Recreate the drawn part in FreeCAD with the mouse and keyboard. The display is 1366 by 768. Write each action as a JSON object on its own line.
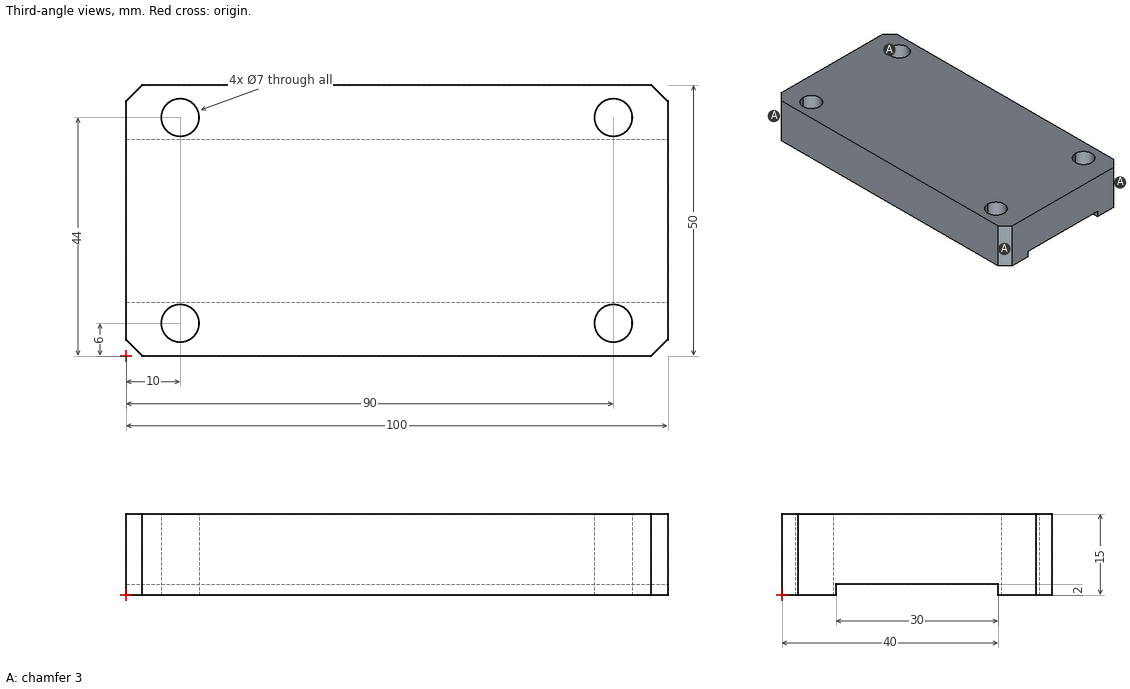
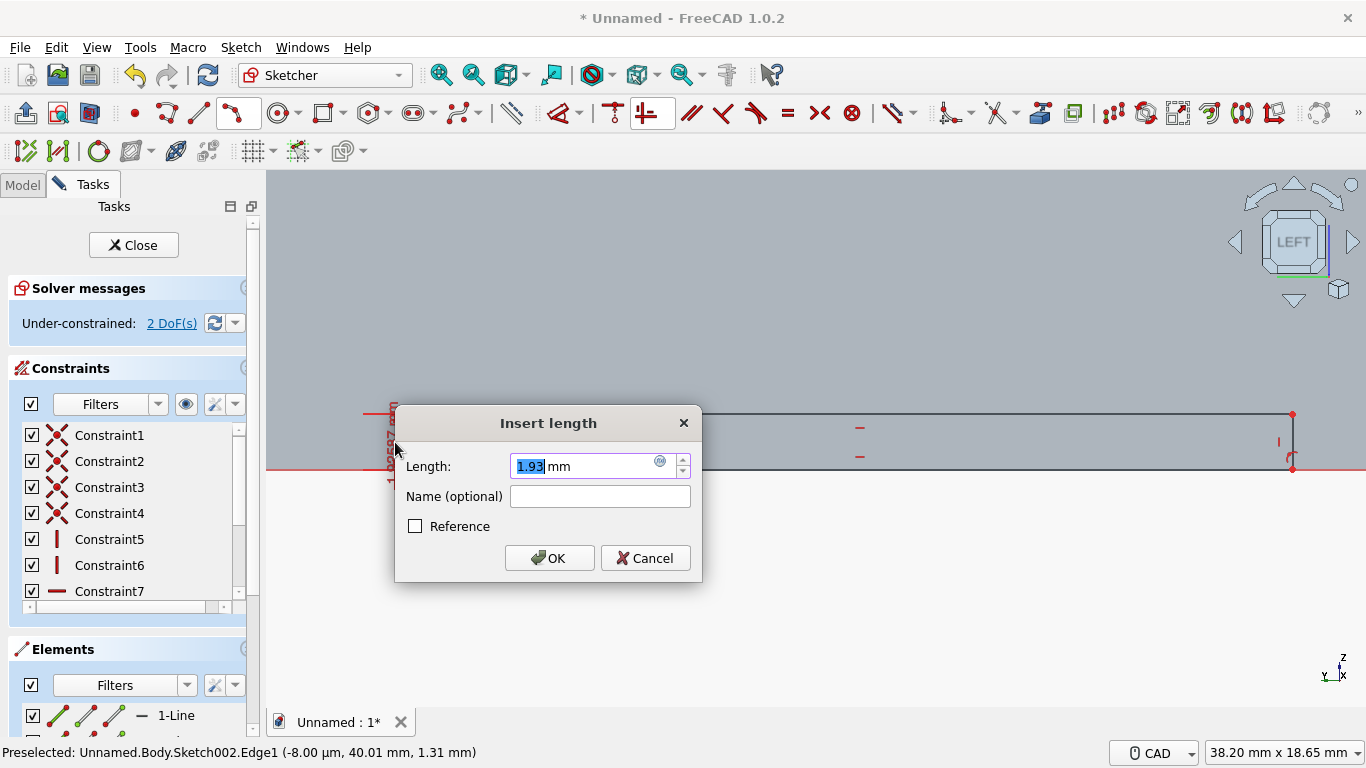
{"action": "type", "text": "2"}
{"action": "key", "text": "Return"}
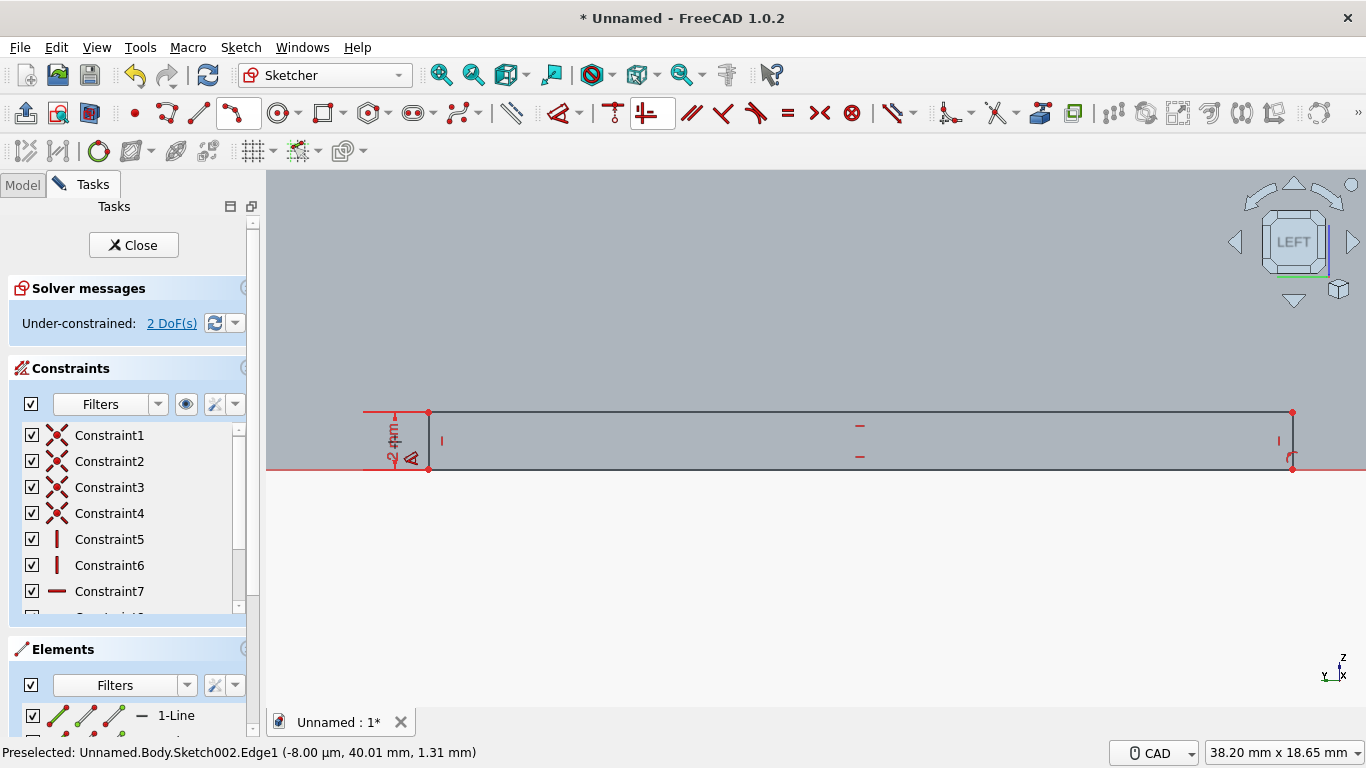
{"action": "left_click", "coordinate": [688, 470]}
{"action": "left_click", "coordinate": [815, 504]}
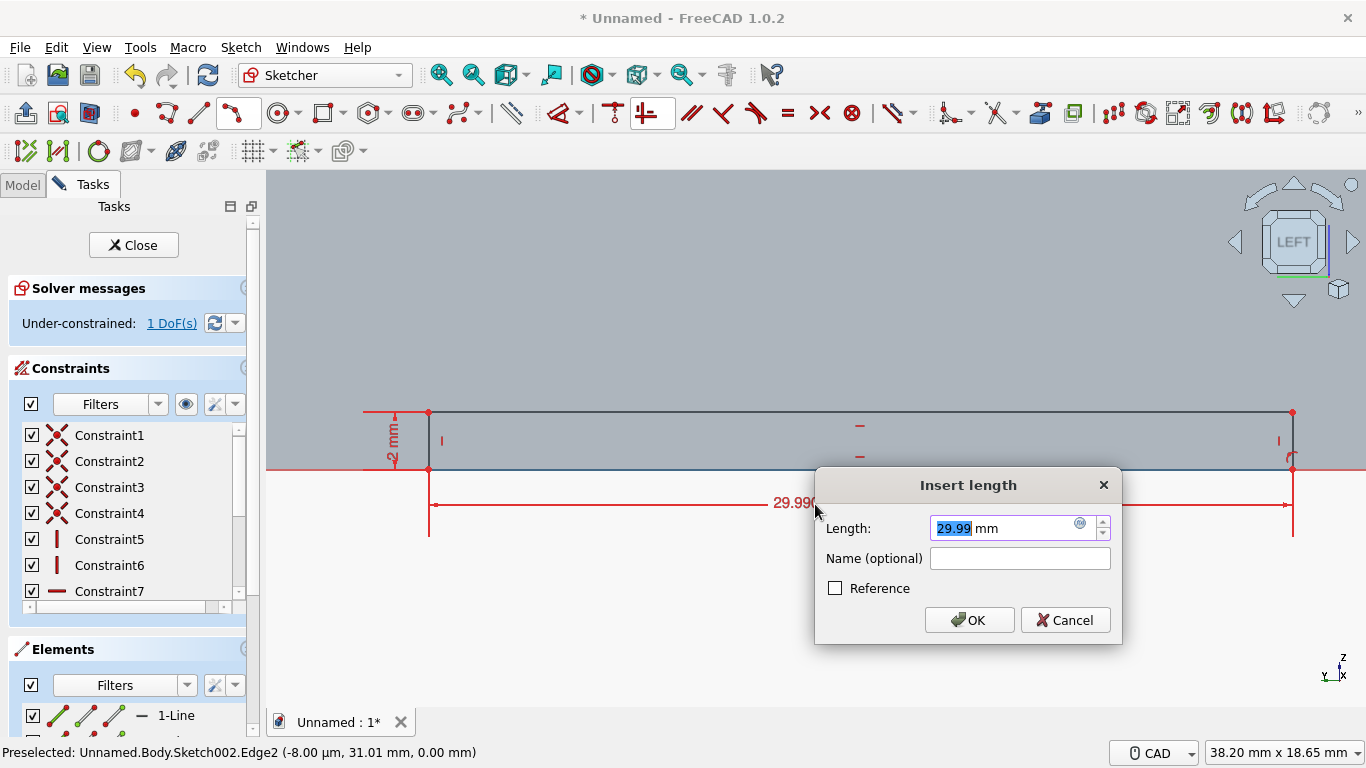
{"action": "type", "text": "30"}
{"action": "key", "text": "Return"}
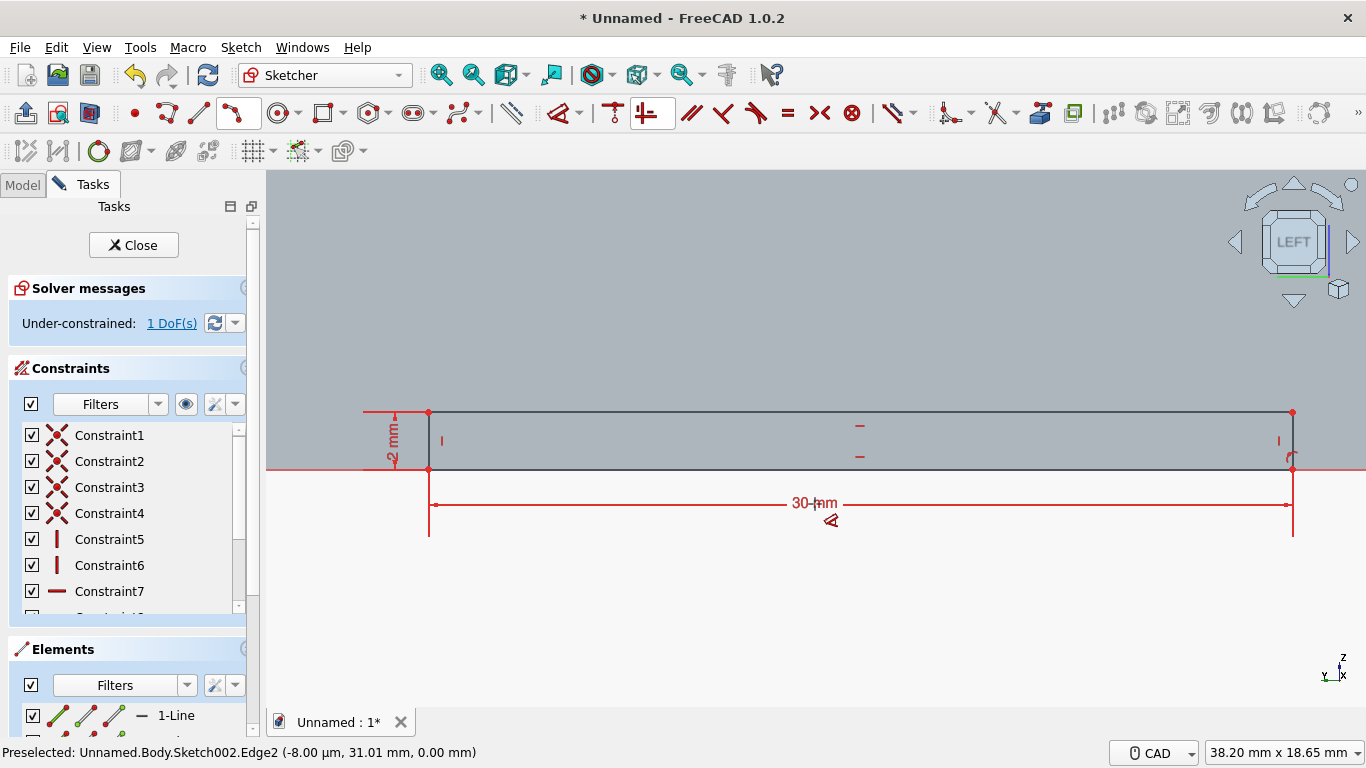
{"action": "left_click", "coordinate": [429, 412]}
{"action": "left_click", "coordinate": [637, 504]}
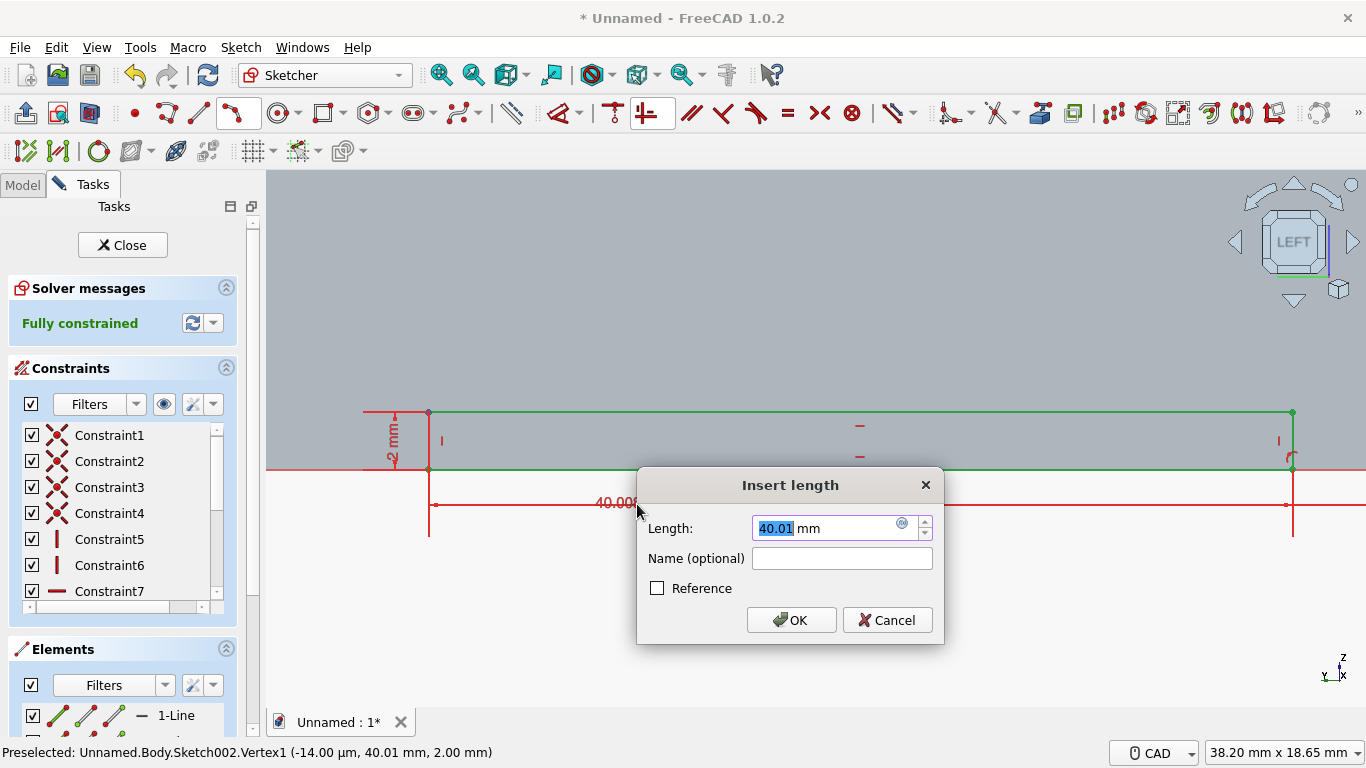
{"action": "type", "text": "40"}
{"action": "key", "text": "Return"}
{"action": "key", "text": "Escape"}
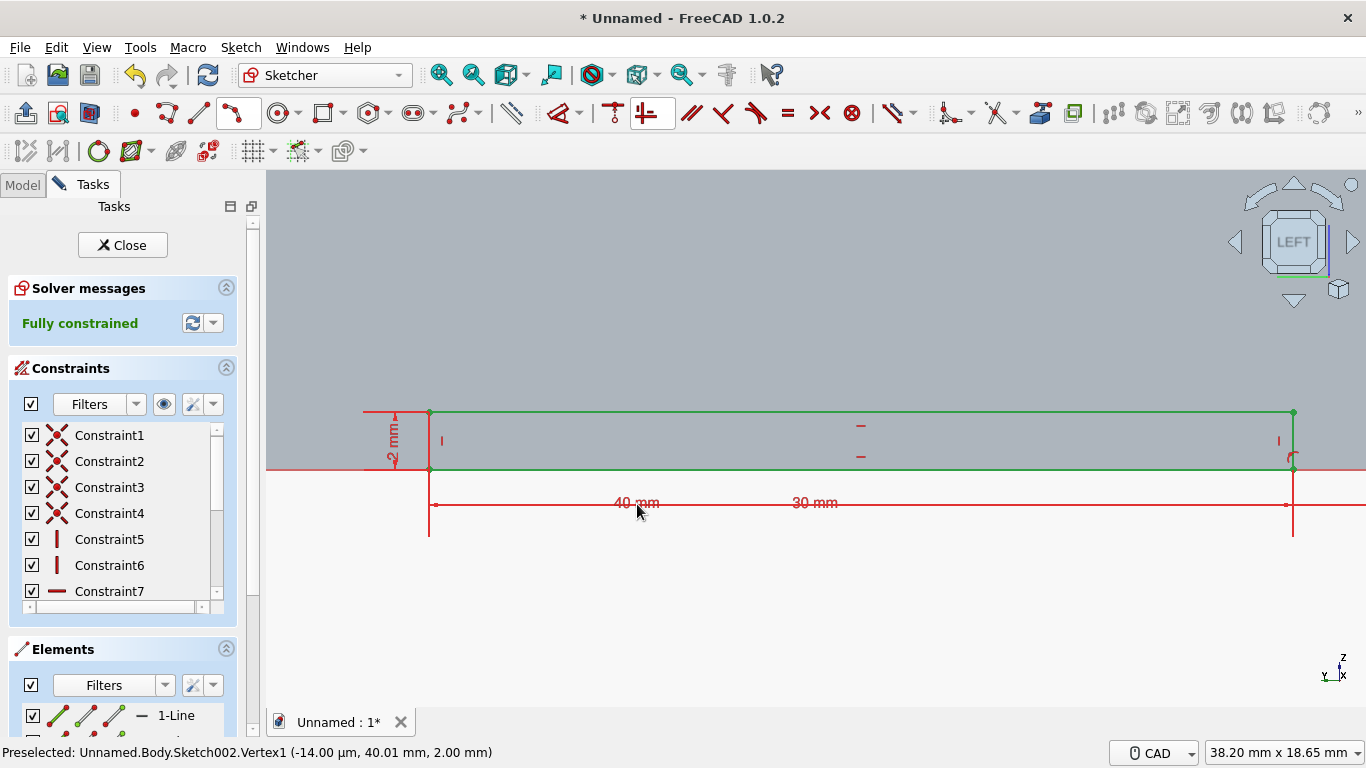
{"action": "left_click", "coordinate": [123, 245]}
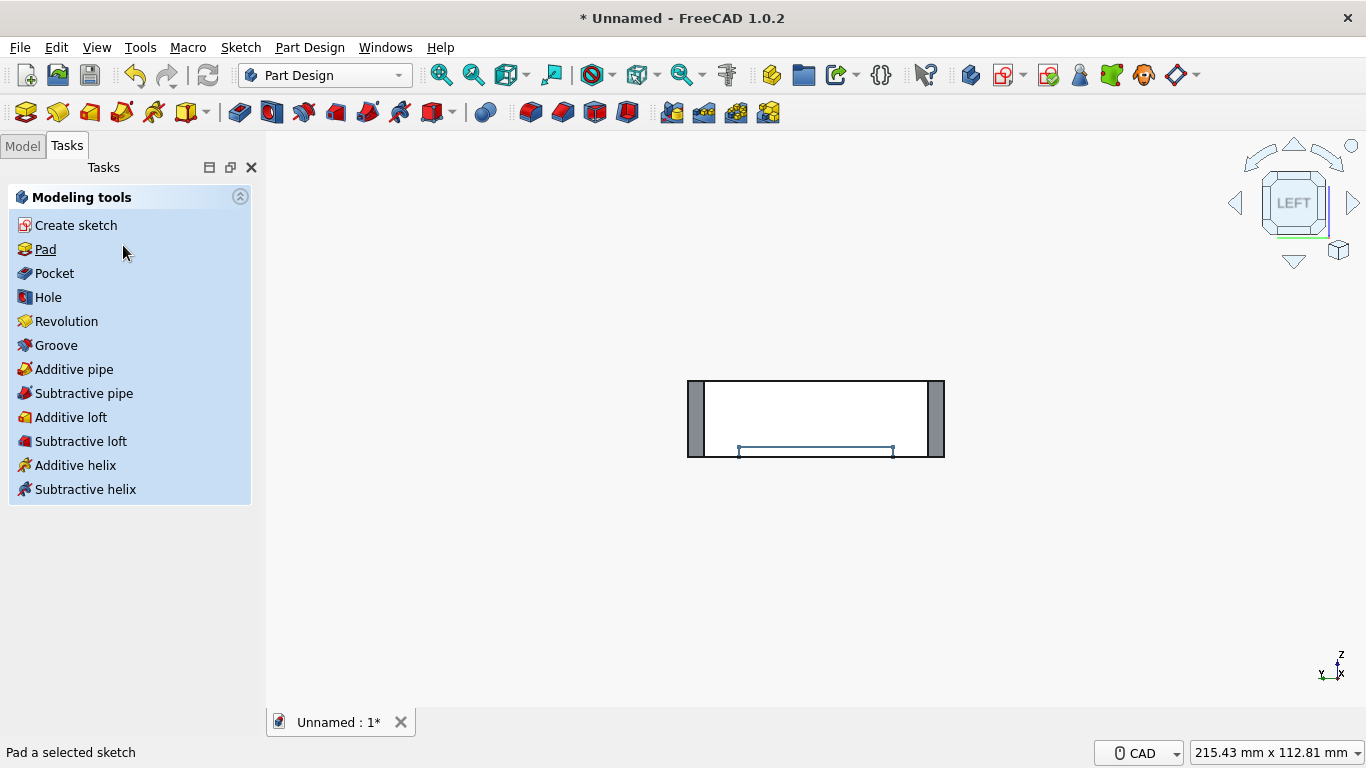
{"action": "left_click", "coordinate": [240, 112]}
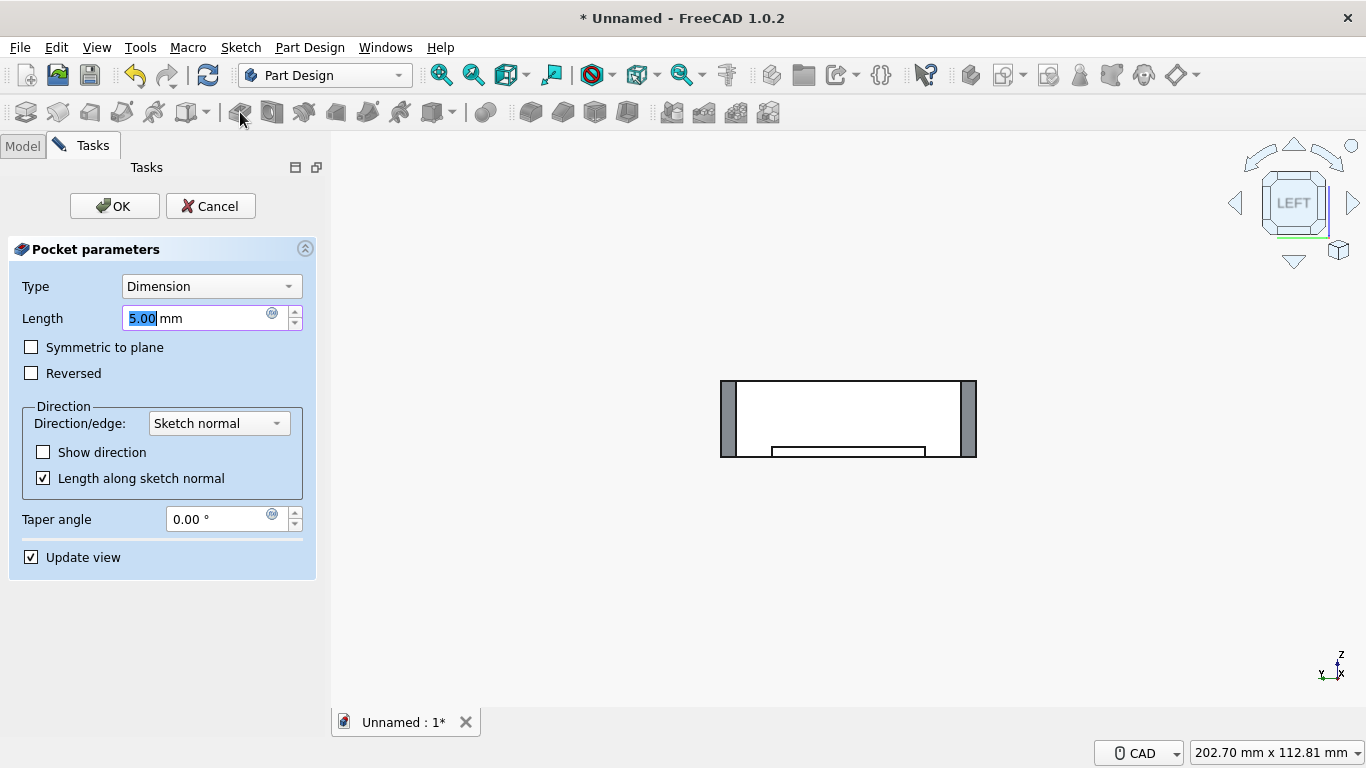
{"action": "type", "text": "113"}
{"action": "key", "text": "Tab"}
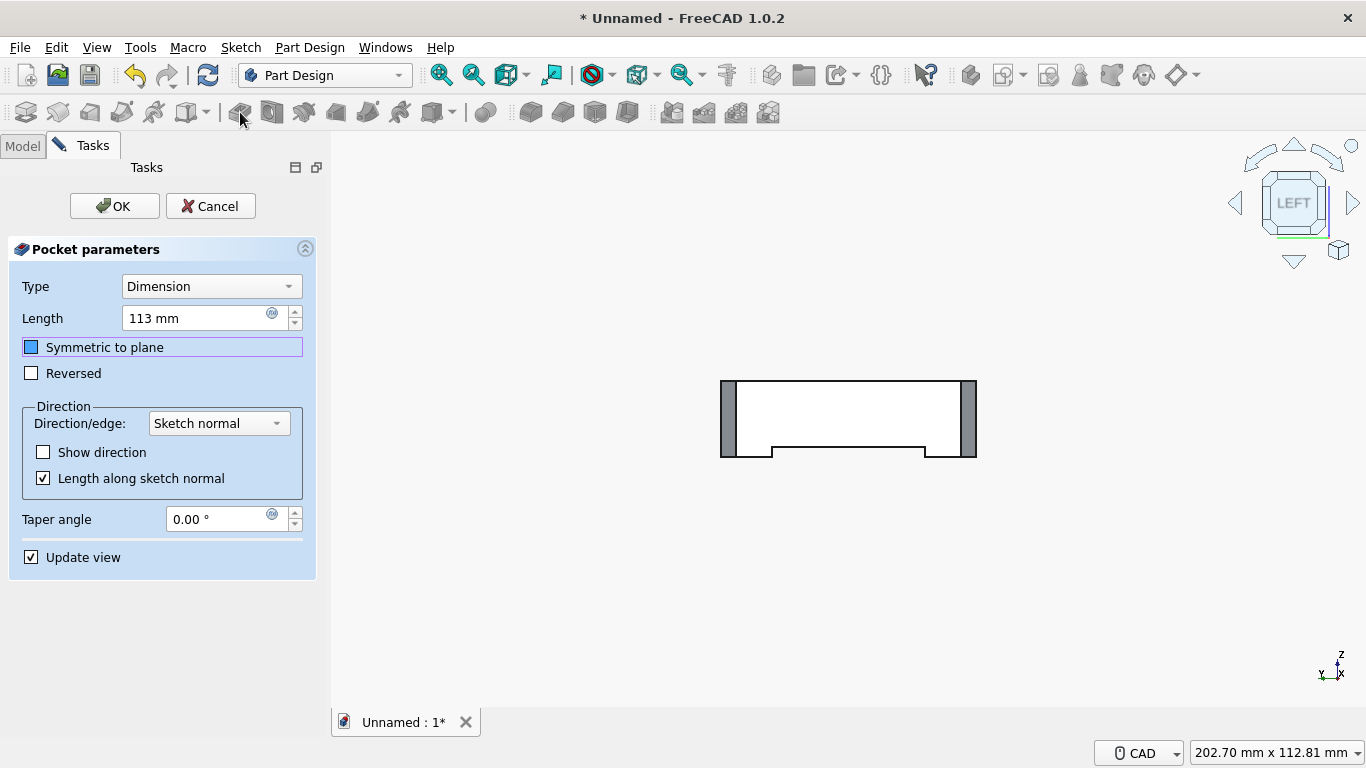
{"action": "left_click", "coordinate": [115, 206]}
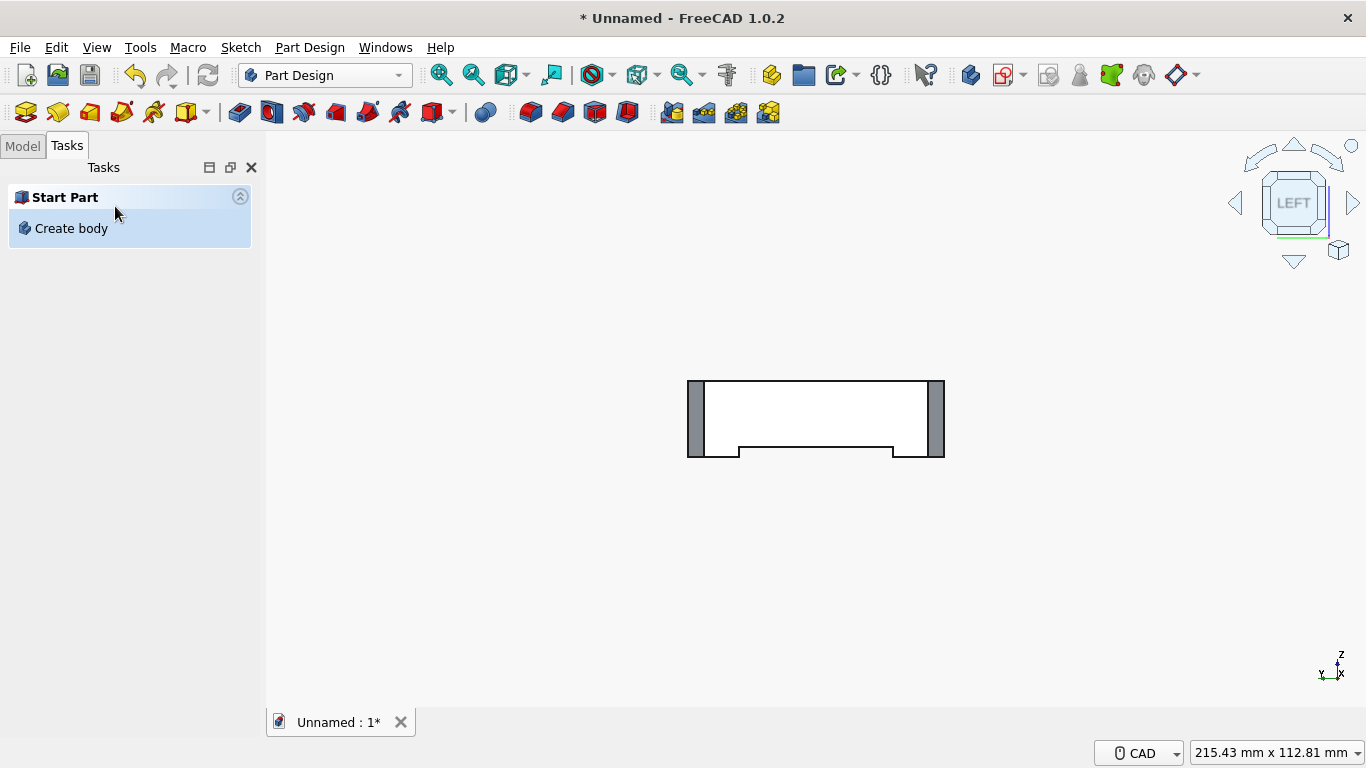
{"action": "key", "text": "0"}